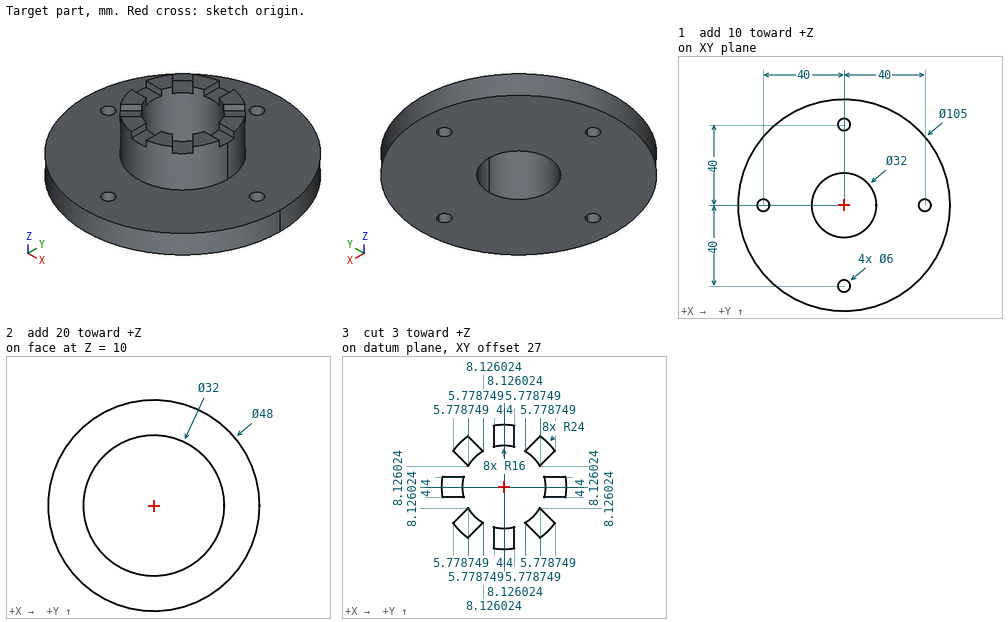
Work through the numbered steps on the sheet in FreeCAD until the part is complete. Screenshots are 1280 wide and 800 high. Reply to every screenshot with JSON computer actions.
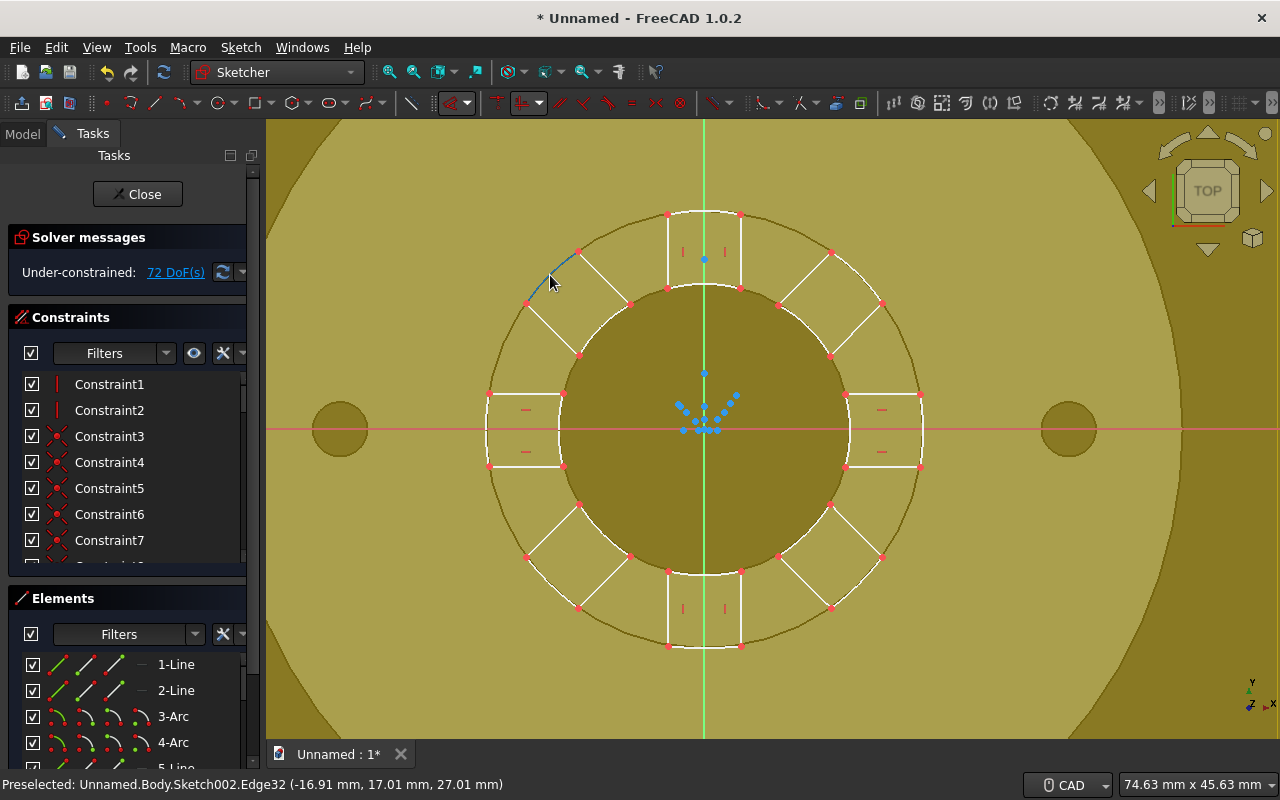
{"action": "left_click", "coordinate": [719, 285]}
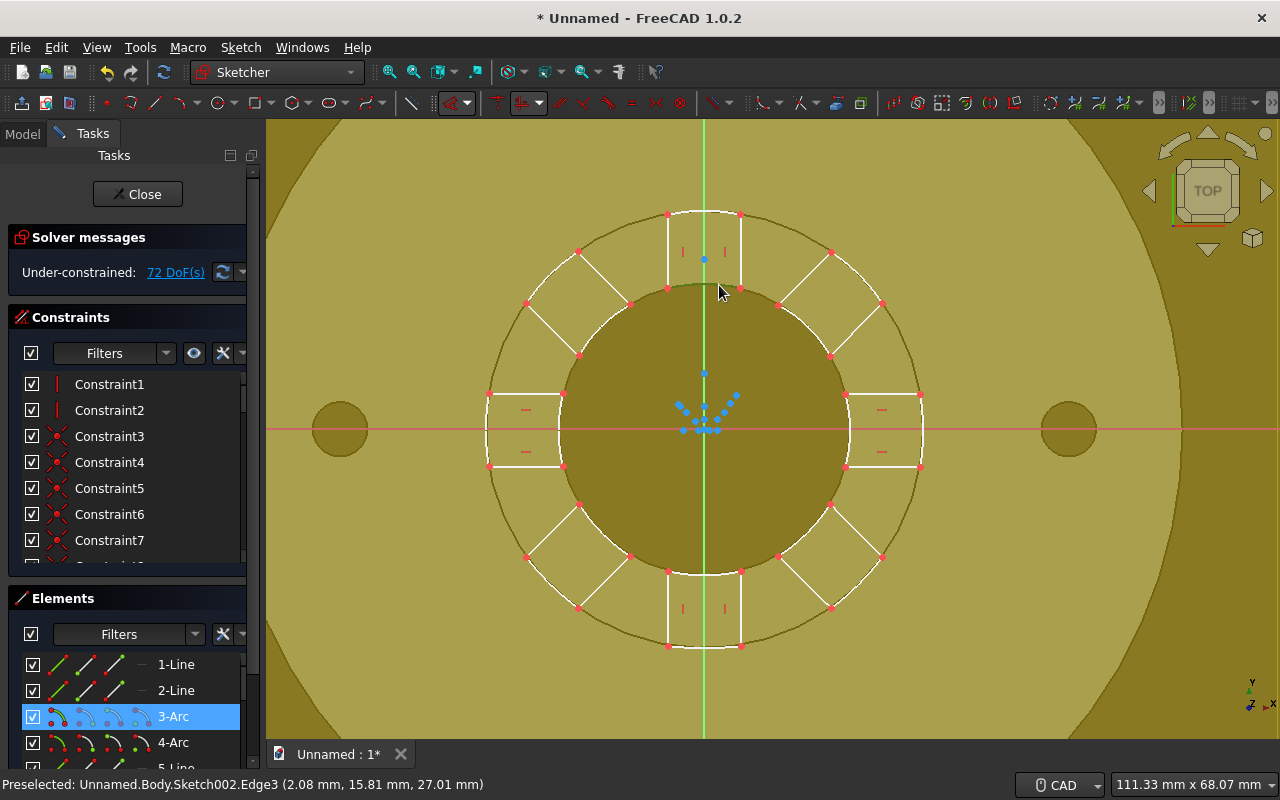
{"action": "left_click", "coordinate": [719, 211]}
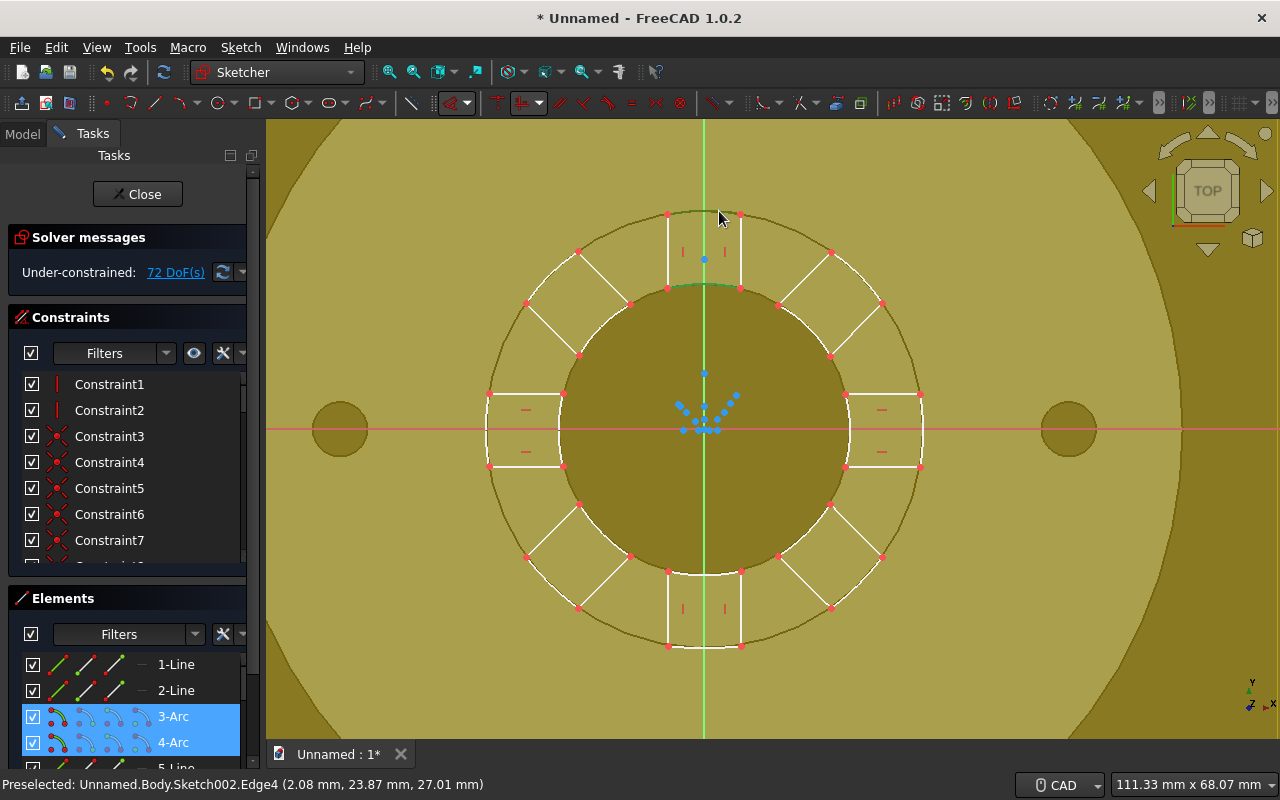
{"action": "left_click", "coordinate": [498, 104]}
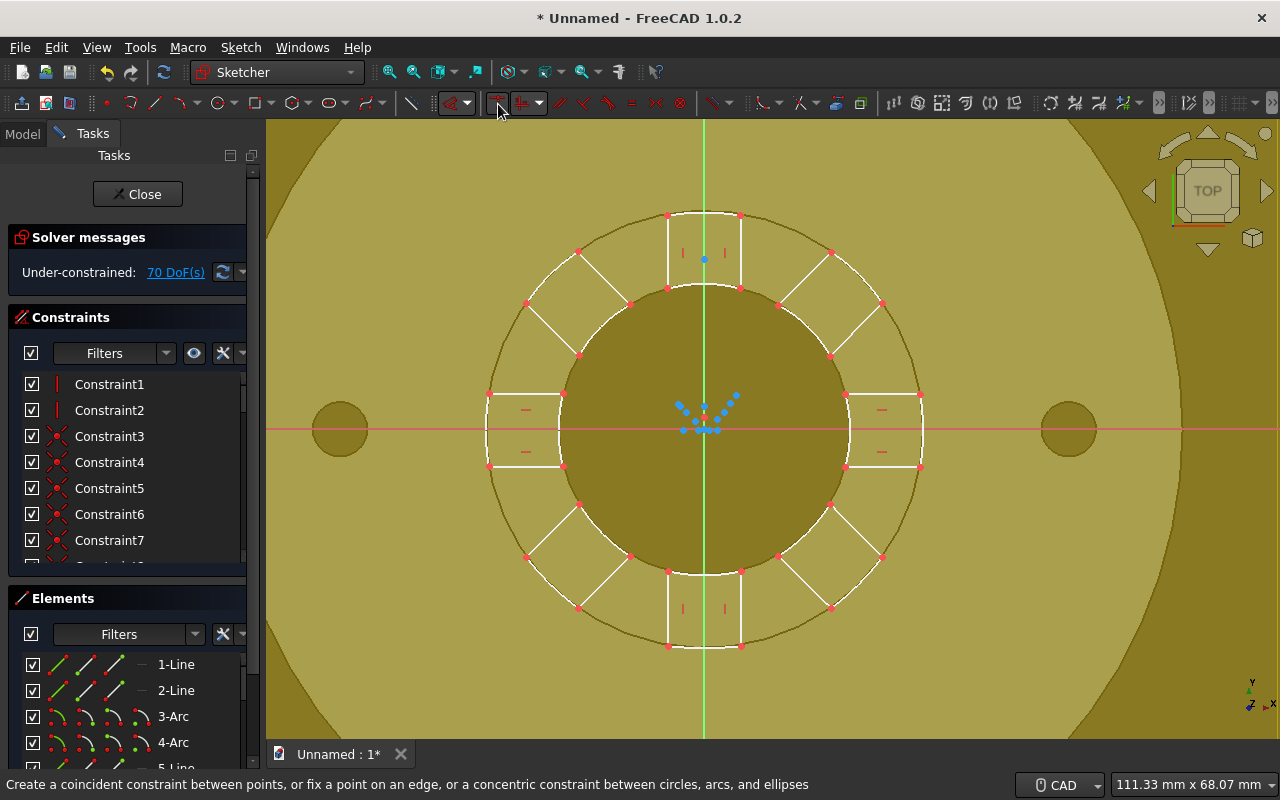
{"action": "left_click", "coordinate": [719, 285]}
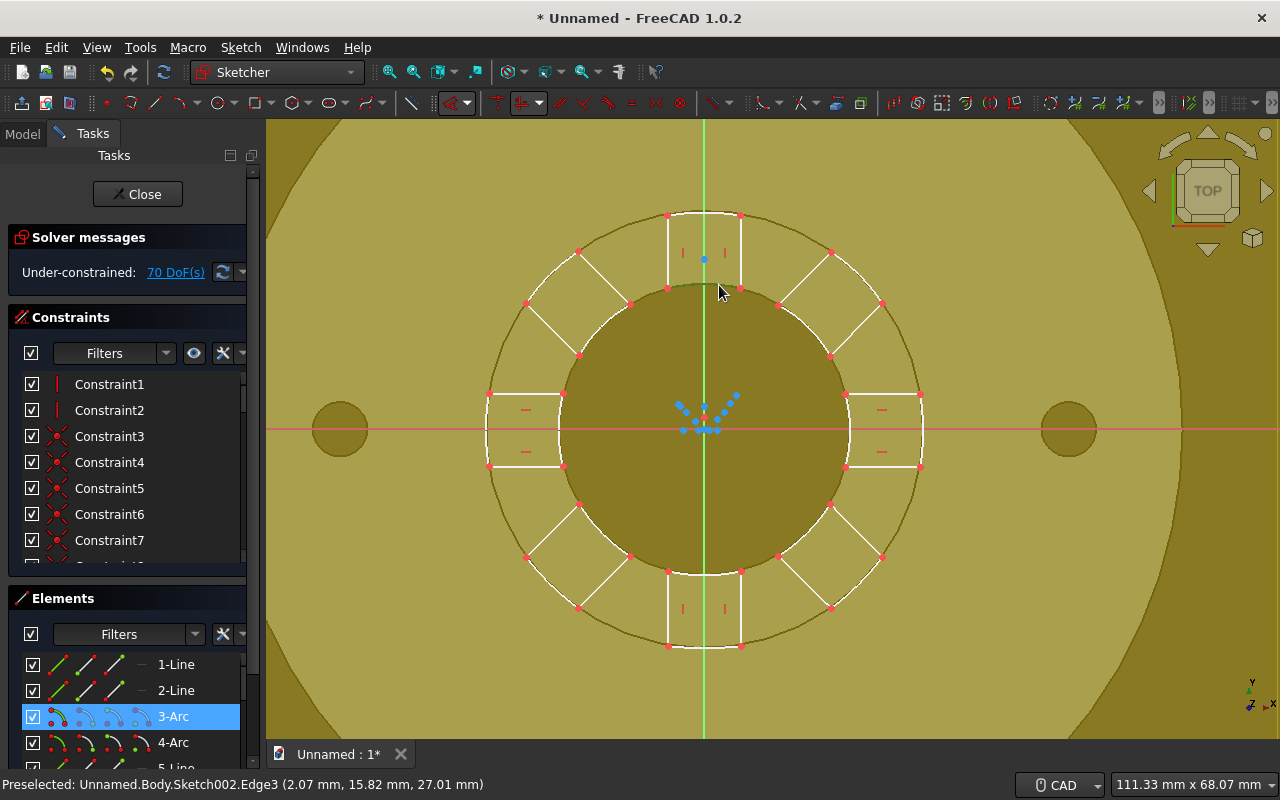
{"action": "left_click", "coordinate": [818, 338]}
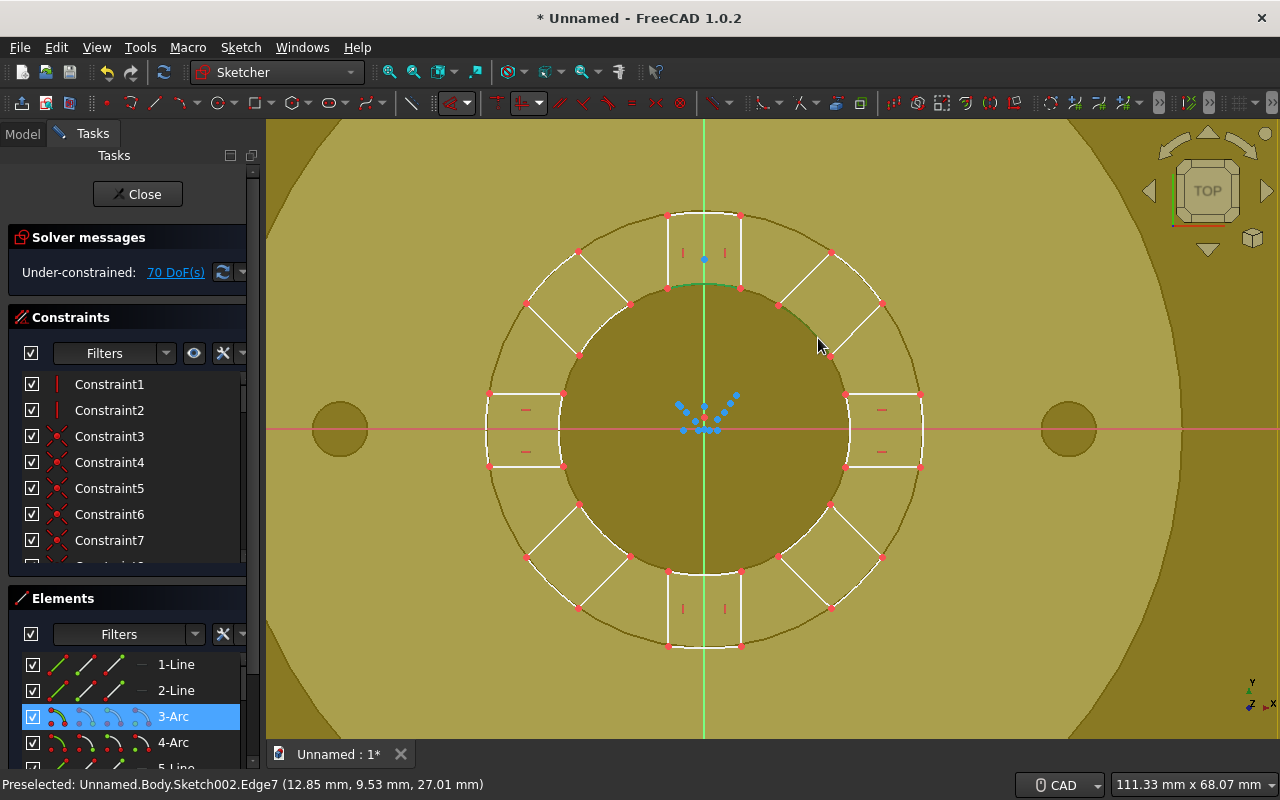
{"action": "left_click", "coordinate": [498, 104]}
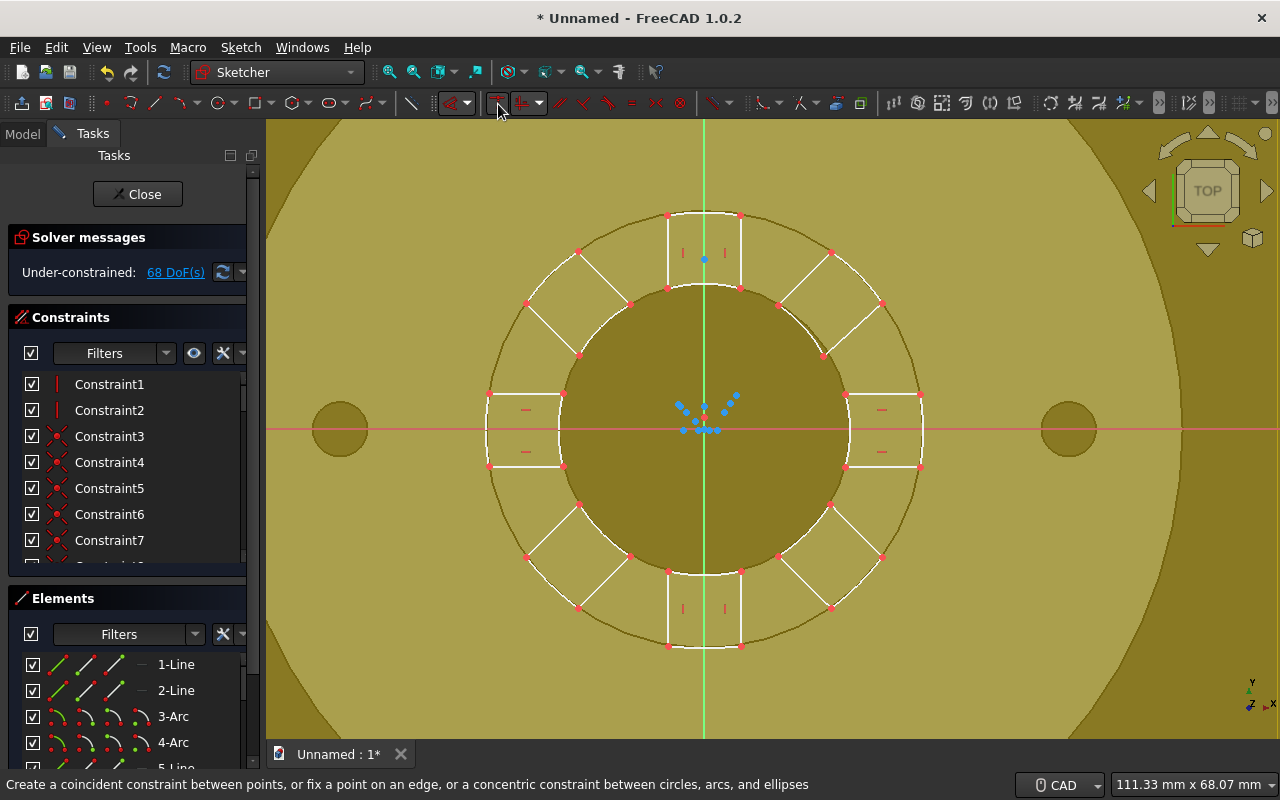
{"action": "left_click", "coordinate": [719, 285]}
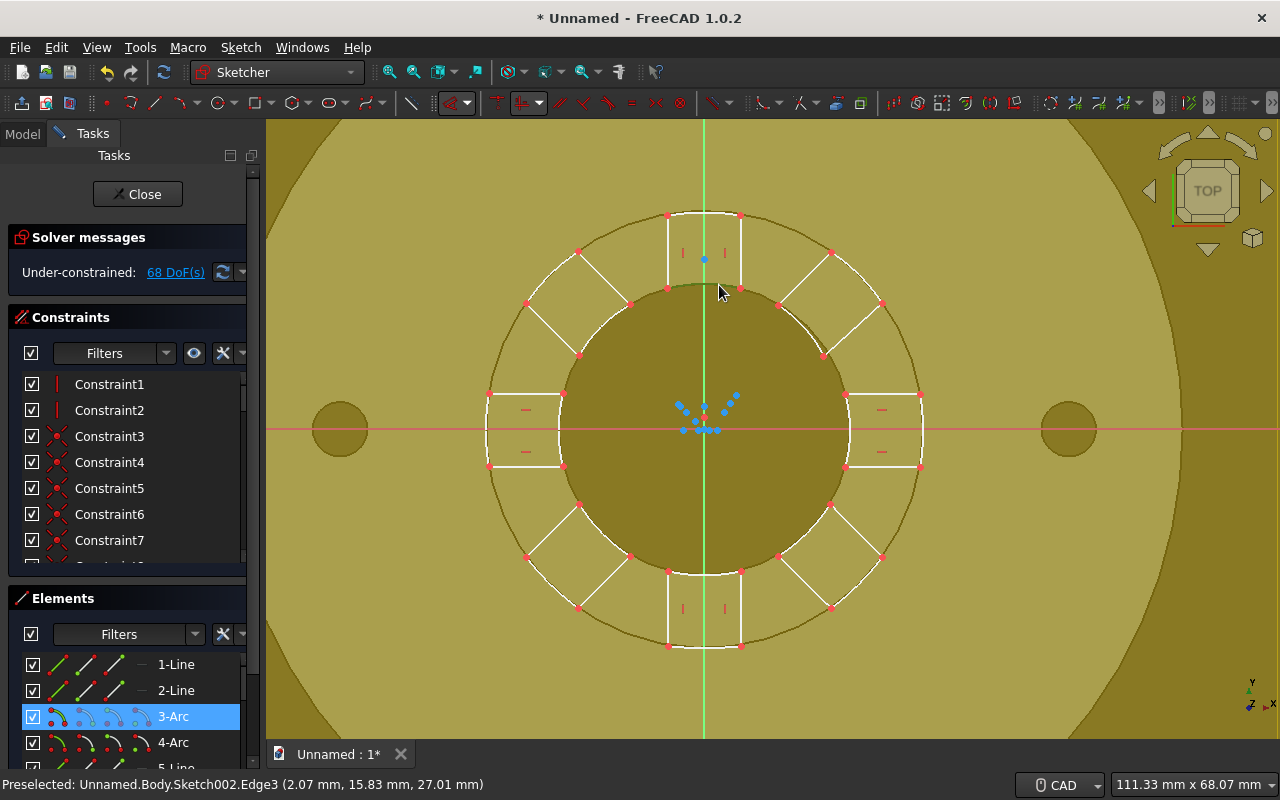
{"action": "left_click", "coordinate": [869, 286]}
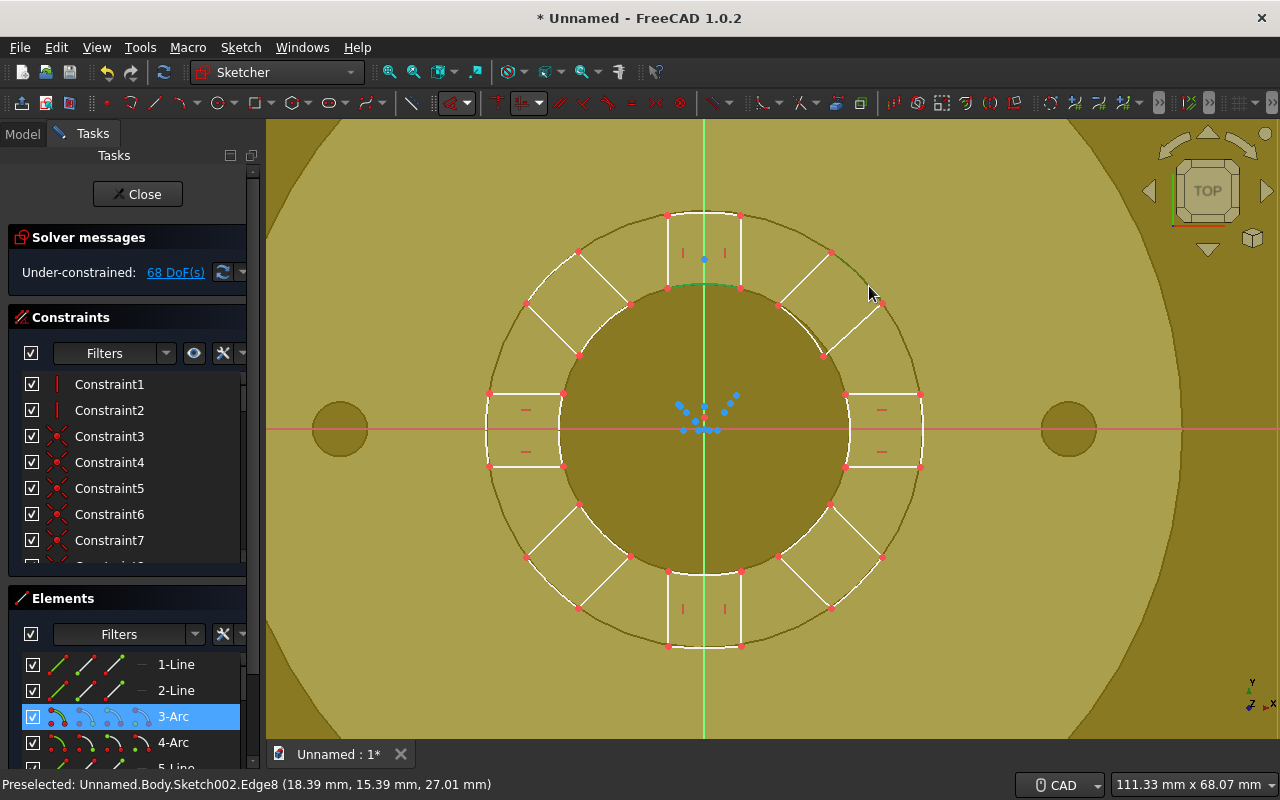
{"action": "left_click", "coordinate": [498, 104]}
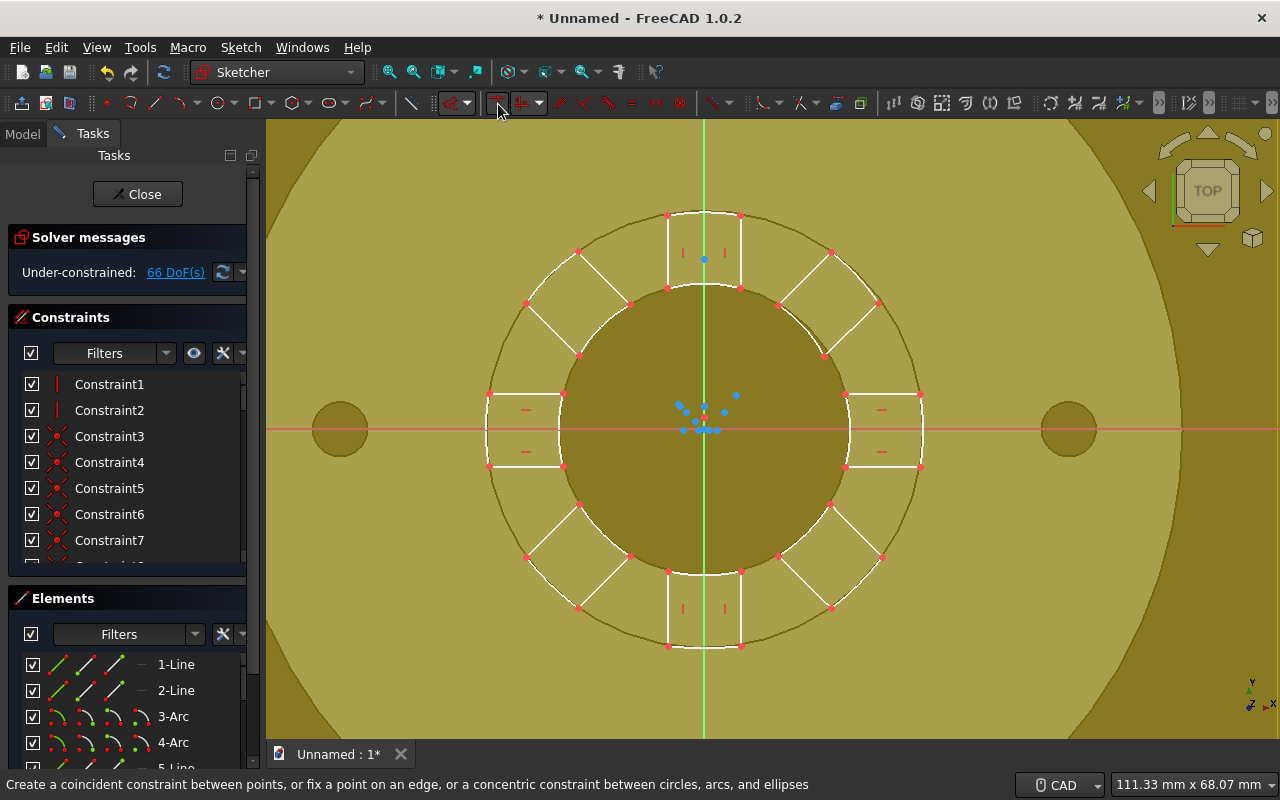
{"action": "left_click", "coordinate": [719, 284]}